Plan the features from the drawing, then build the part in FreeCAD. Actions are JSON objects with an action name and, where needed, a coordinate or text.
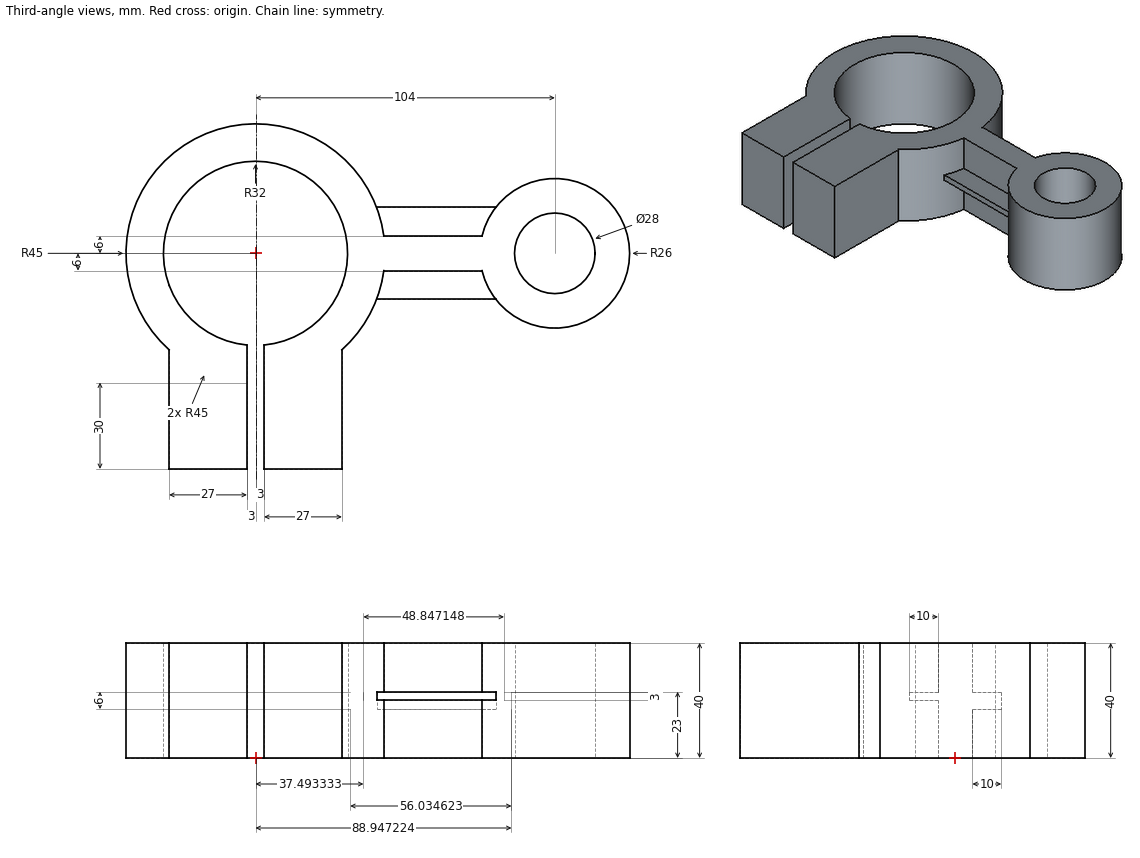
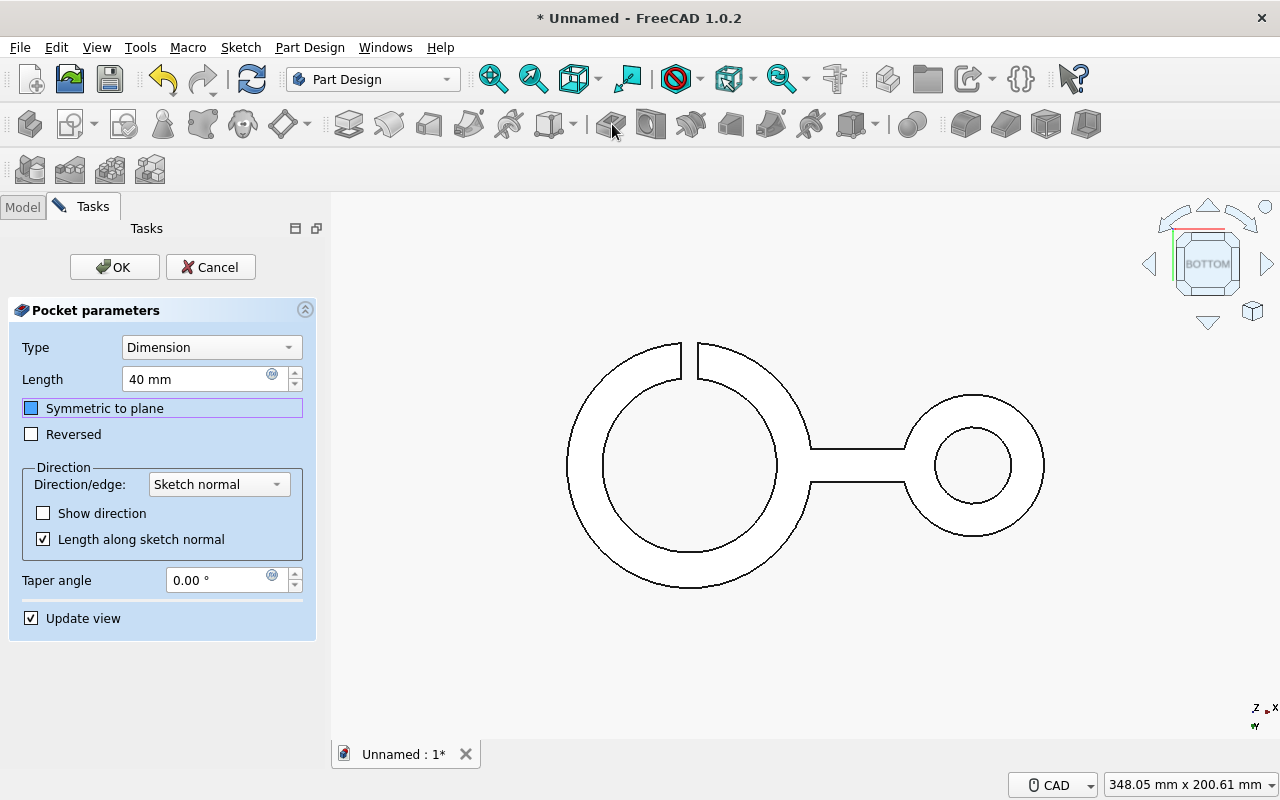
{"action": "left_click", "coordinate": [115, 267]}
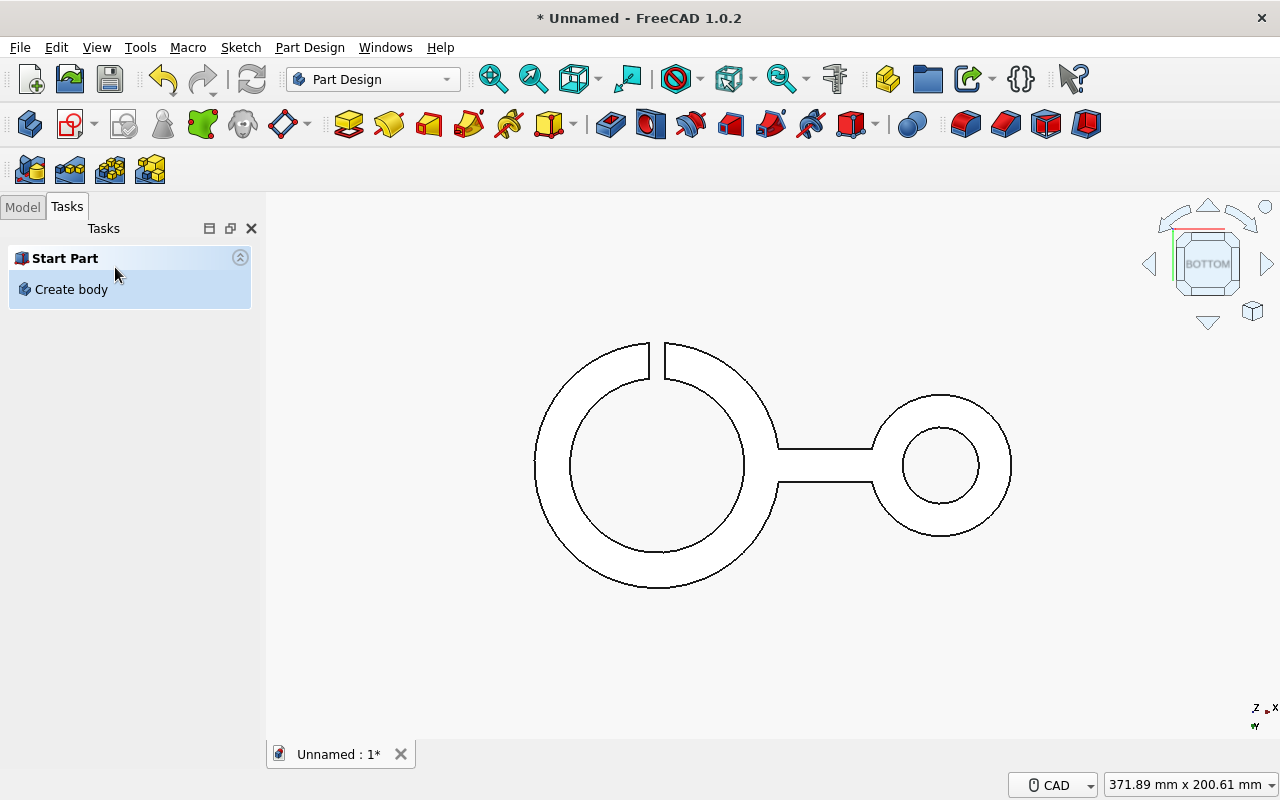
{"action": "left_click", "coordinate": [773, 465]}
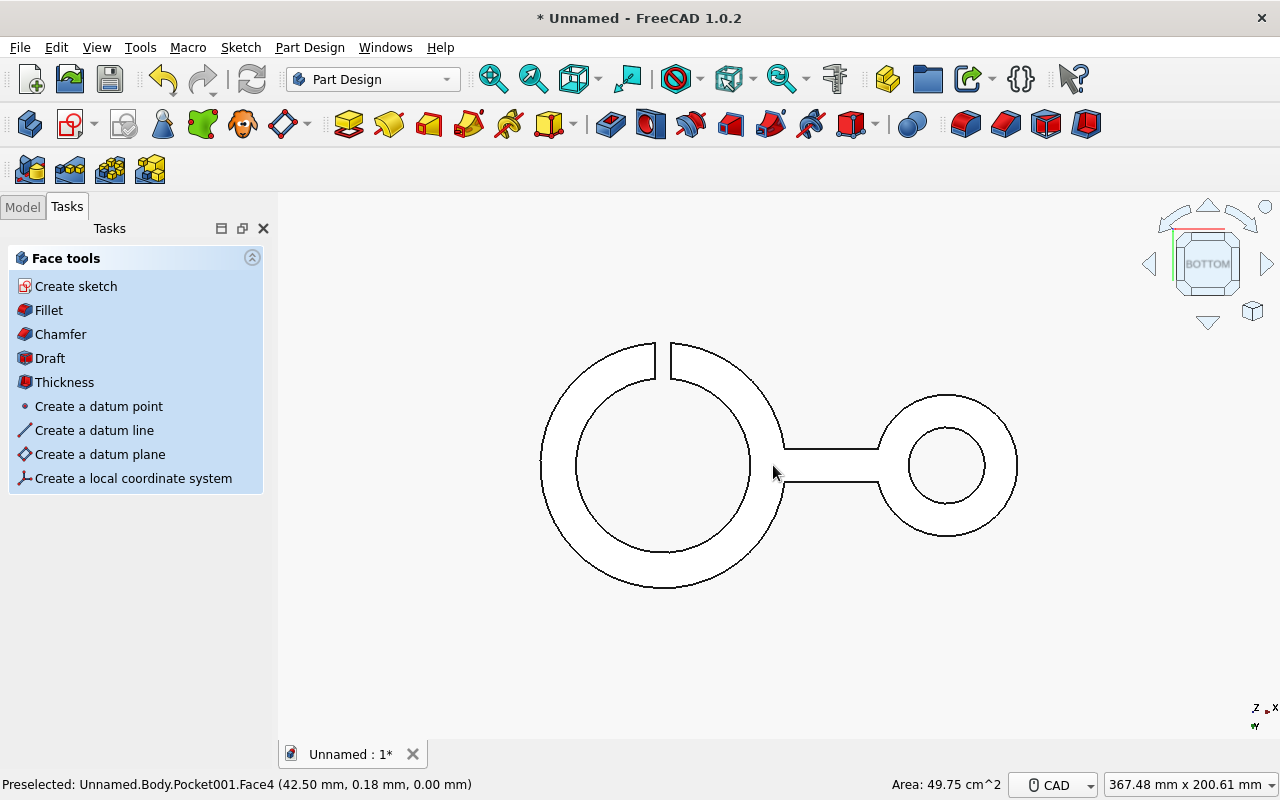
{"action": "left_click", "coordinate": [70, 124]}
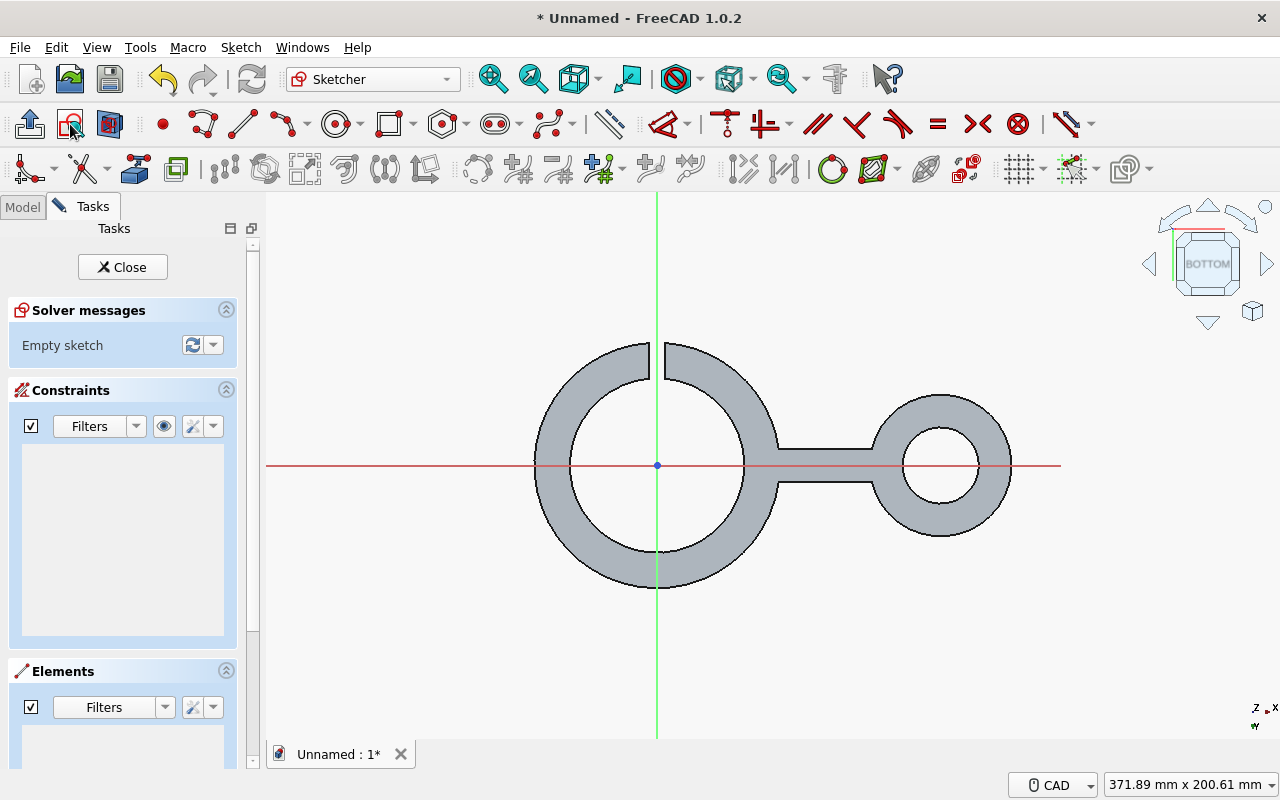
{"action": "scroll", "coordinate": [599, 239], "scroll_direction": "up", "scroll_amount": 3}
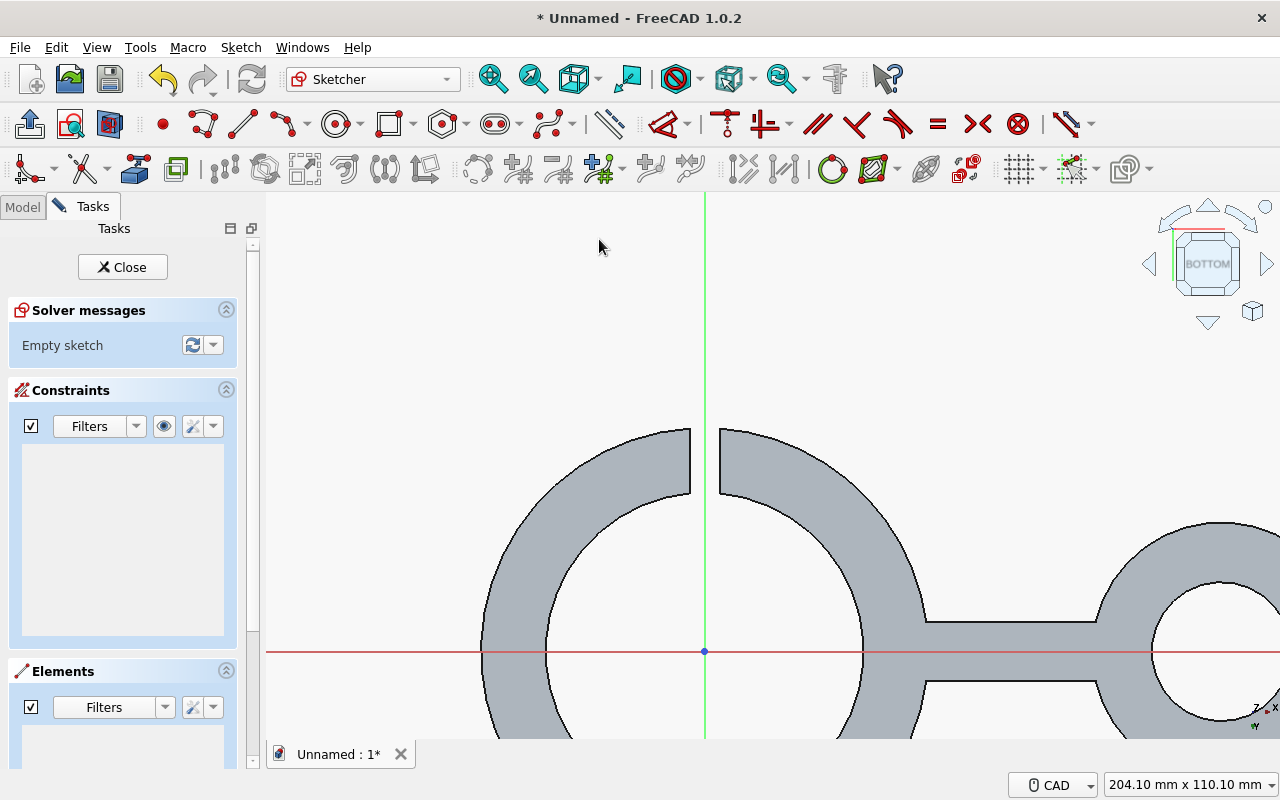
{"action": "key", "text": "g m"}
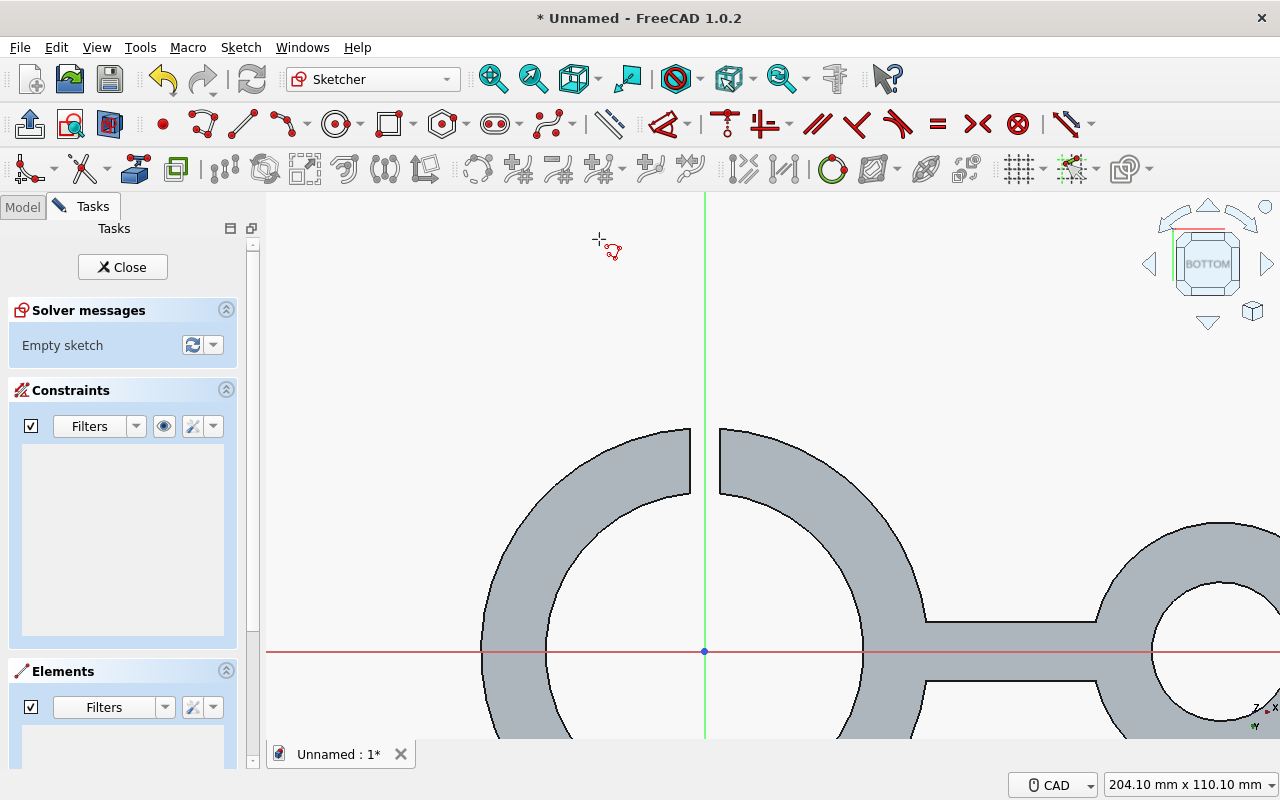
{"action": "left_click", "coordinate": [556, 485]}
{"action": "left_click", "coordinate": [556, 280]}
{"action": "left_click", "coordinate": [690, 280]}
{"action": "left_click", "coordinate": [690, 429]}
{"action": "right_click", "coordinate": [690, 429]}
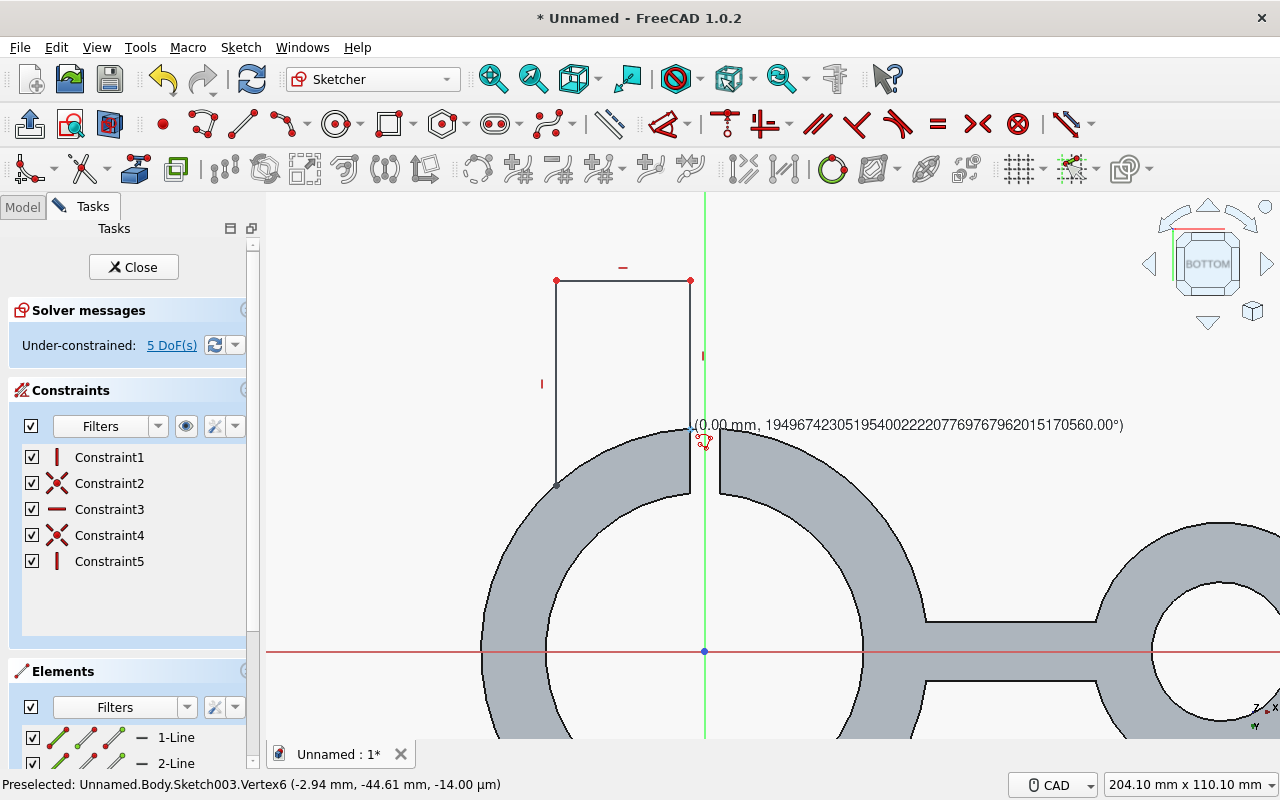
{"action": "key", "text": "g 3 a"}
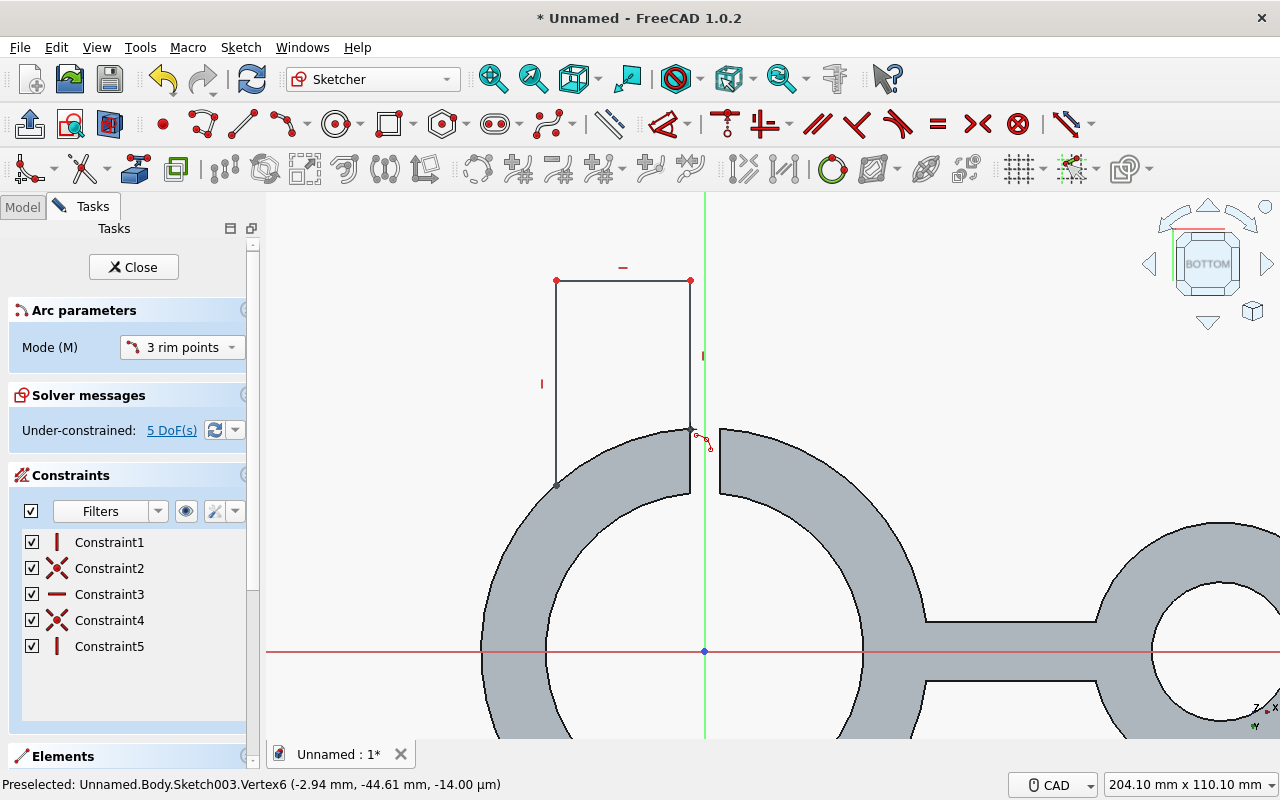
{"action": "left_click", "coordinate": [690, 430]}
{"action": "left_click", "coordinate": [556, 486]}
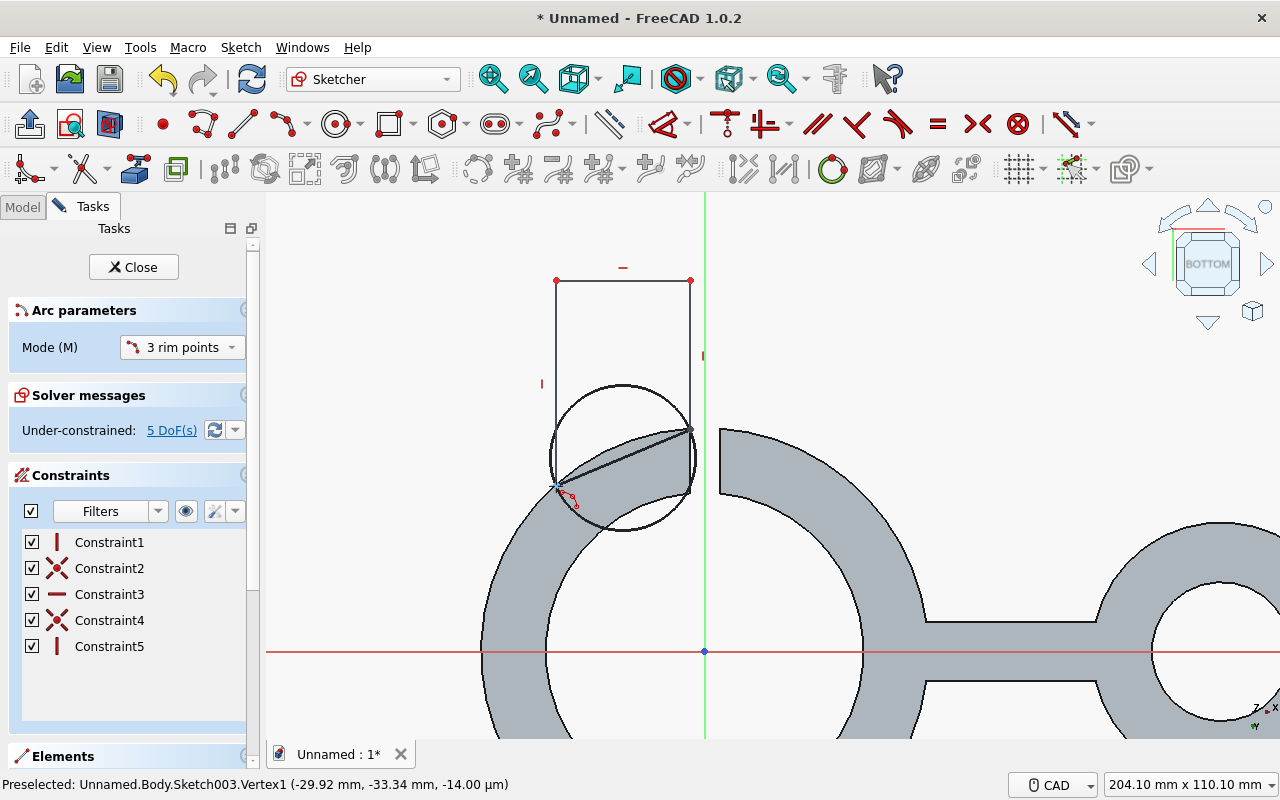
{"action": "scroll", "coordinate": [618, 446], "scroll_direction": "up", "scroll_amount": 2}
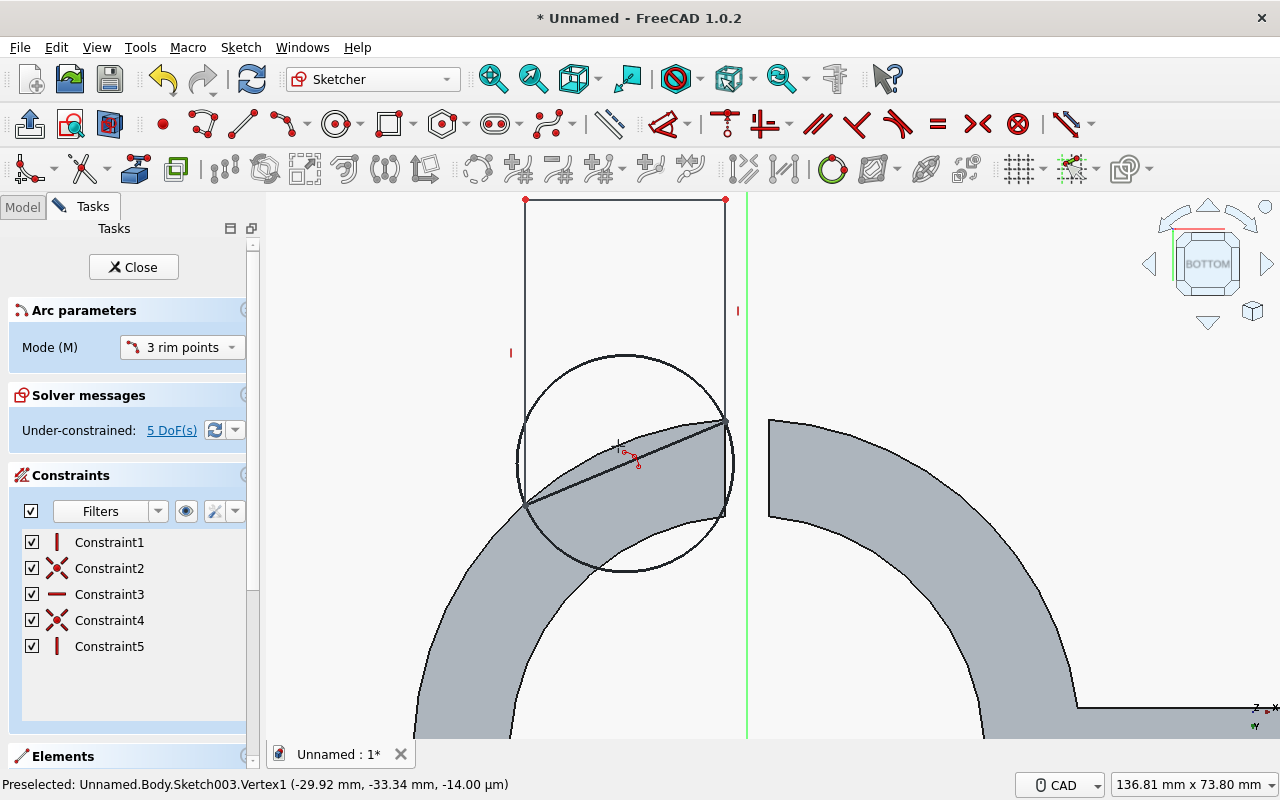
{"action": "left_click", "coordinate": [618, 445]}